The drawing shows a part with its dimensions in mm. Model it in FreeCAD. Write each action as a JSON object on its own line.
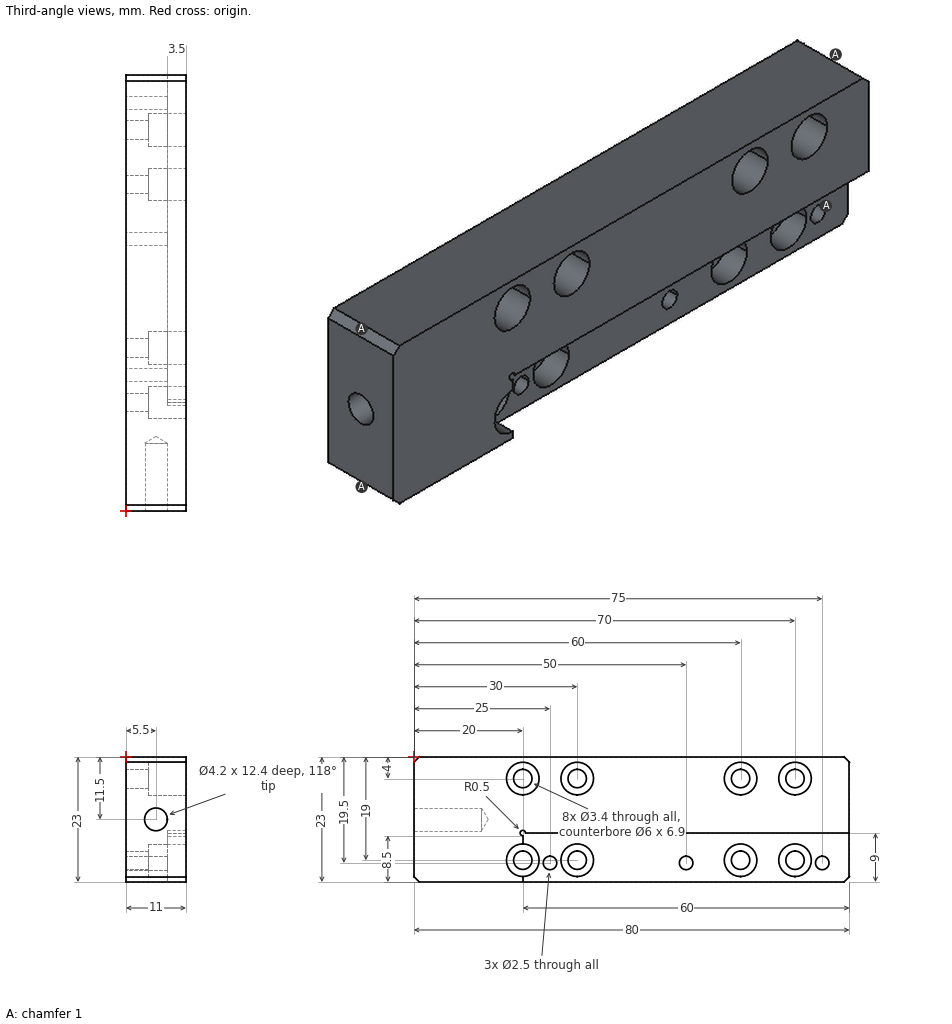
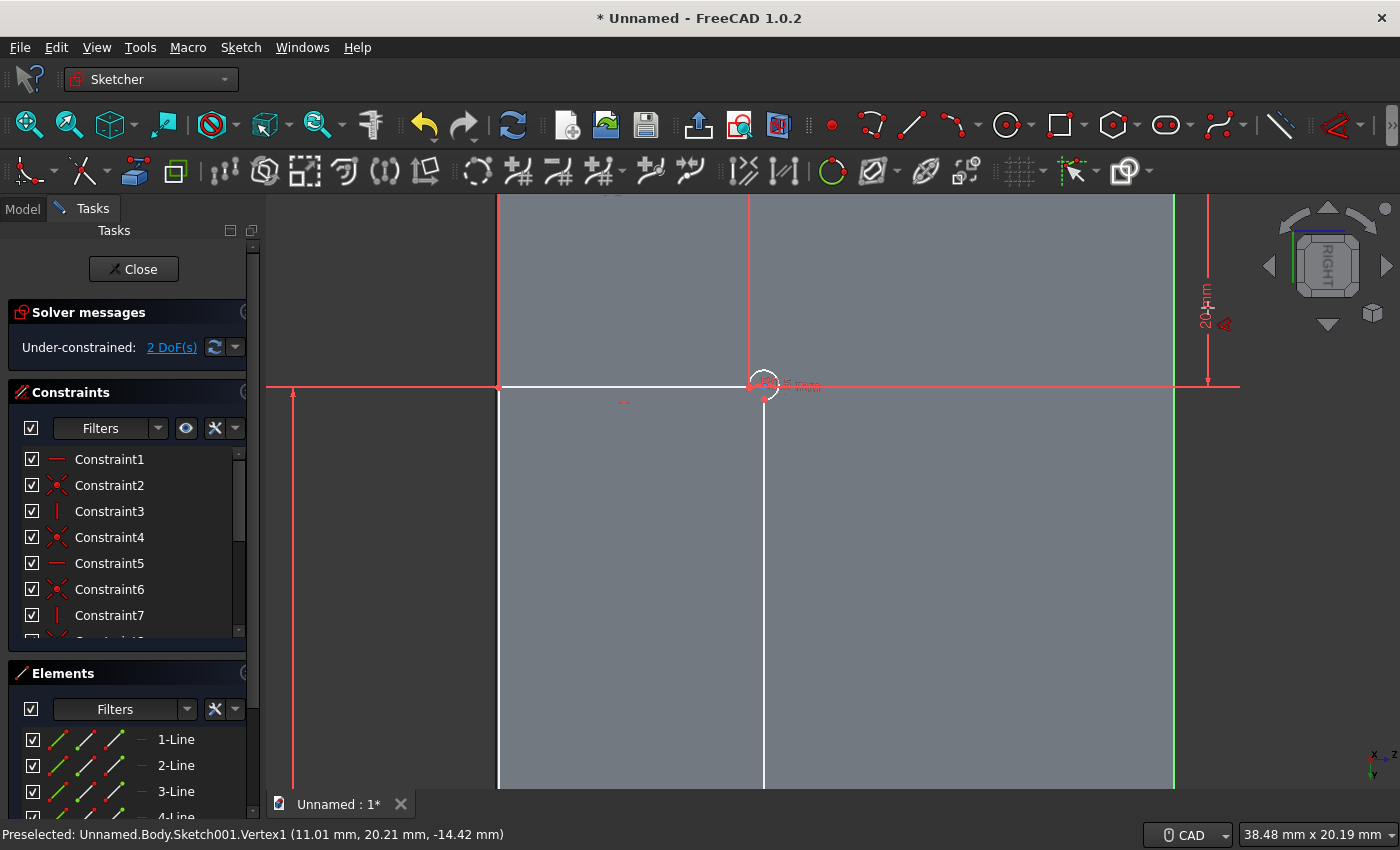
{"action": "scroll", "coordinate": [750, 395], "scroll_direction": "down", "scroll_amount": 9}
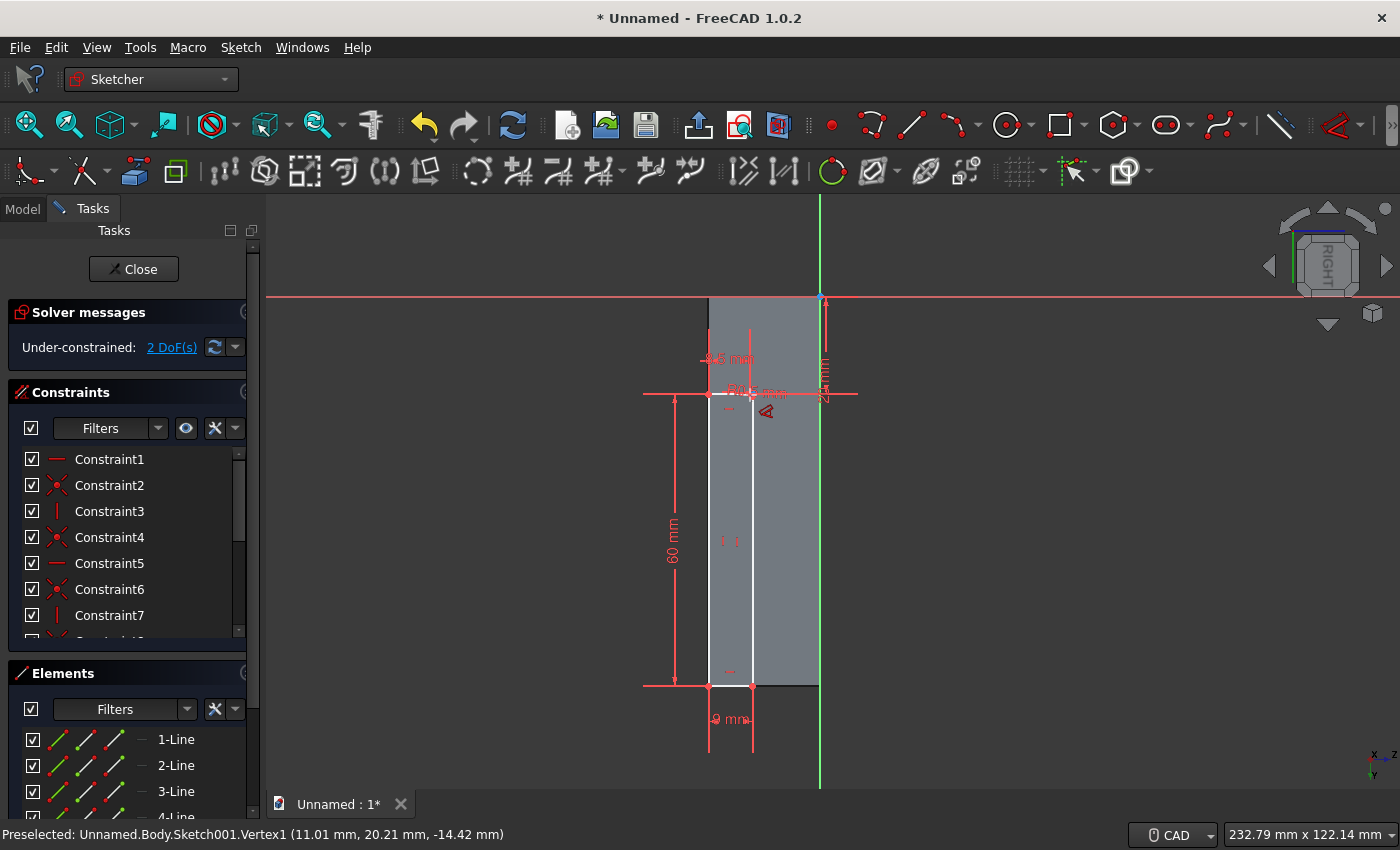
{"action": "left_click", "coordinate": [709, 394]}
{"action": "left_click", "coordinate": [765, 263]}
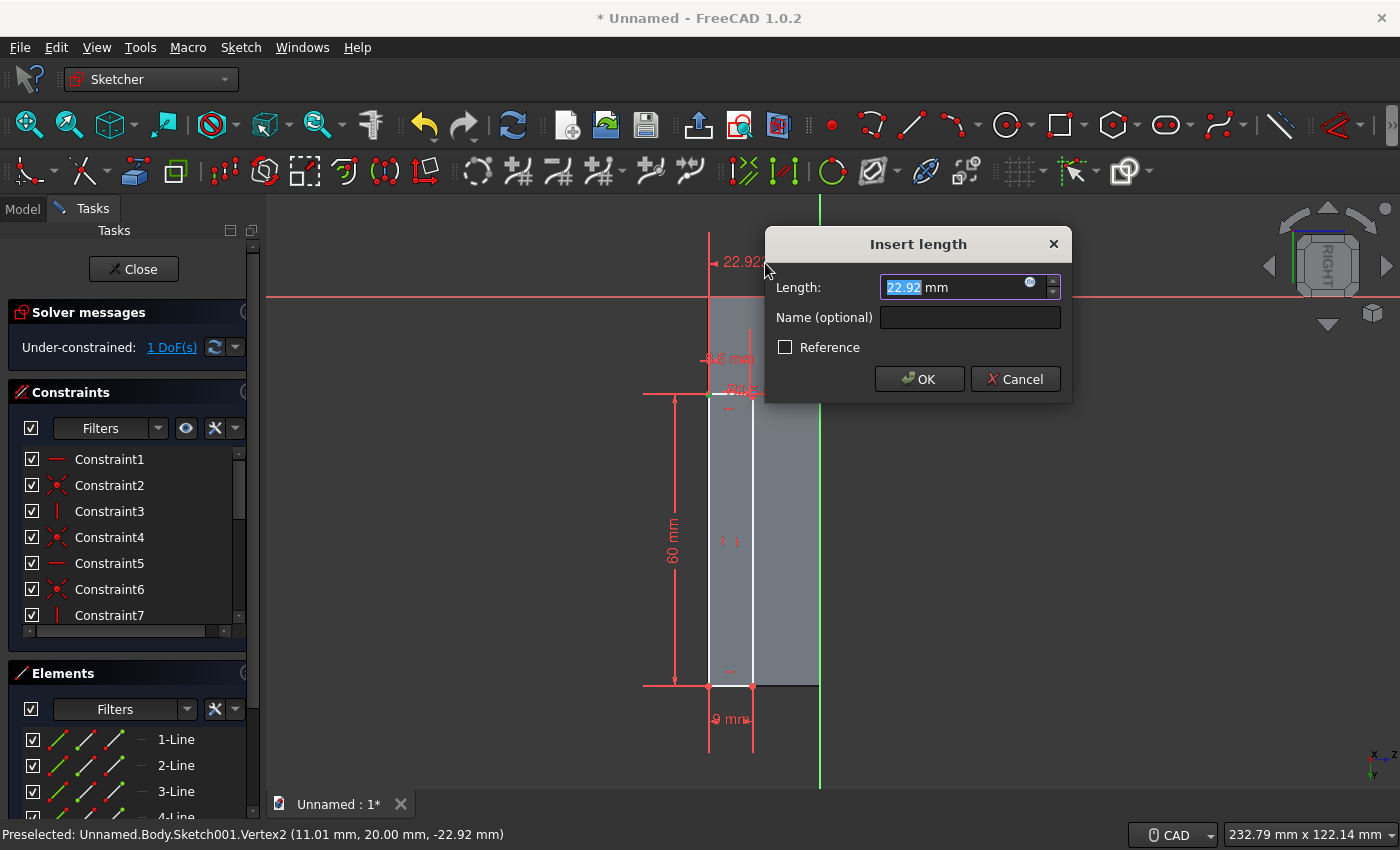
{"action": "type", "text": "23"}
{"action": "key", "text": "Return"}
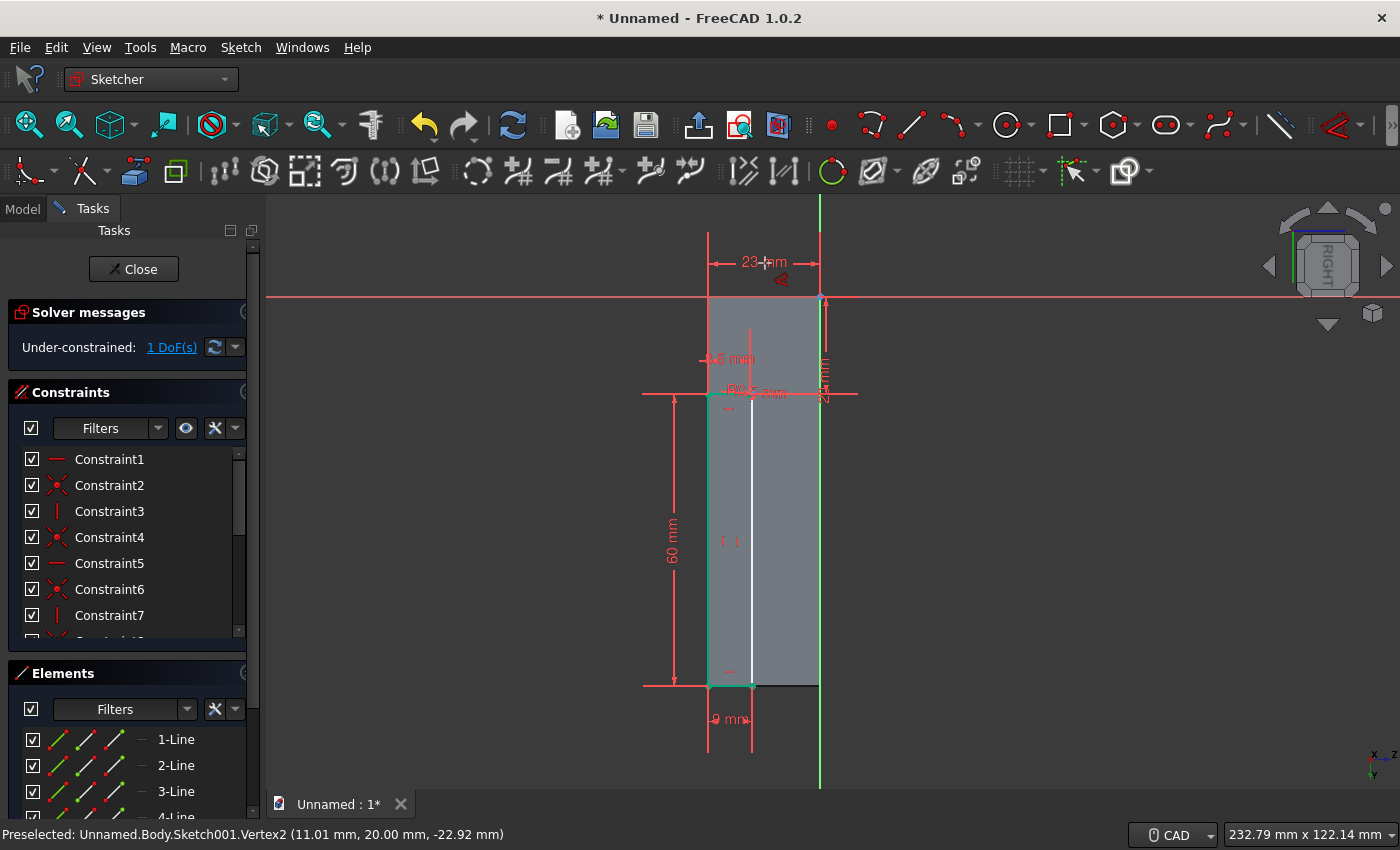
{"action": "scroll", "coordinate": [752, 394], "scroll_direction": "up", "scroll_amount": 9}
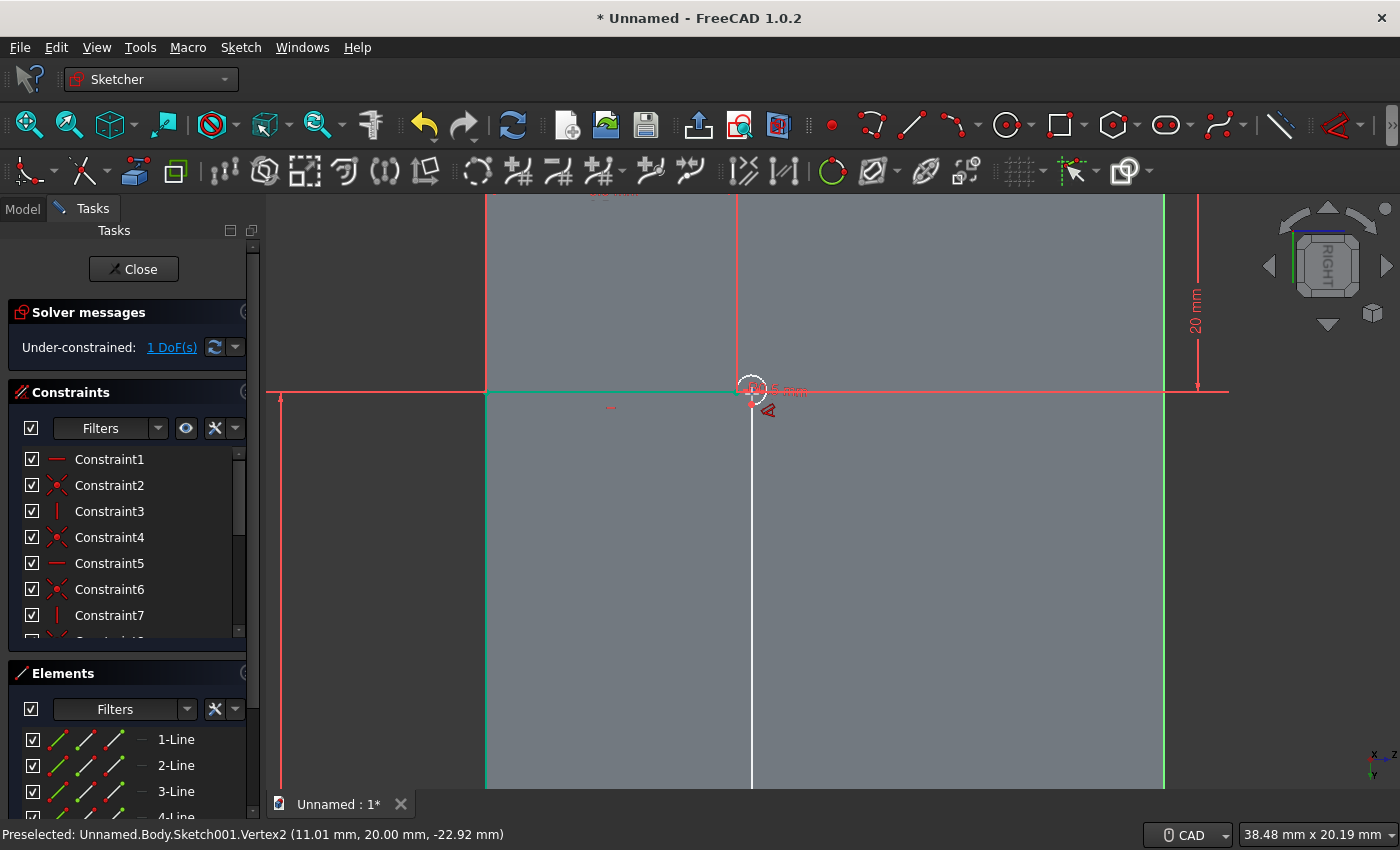
{"action": "left_click", "coordinate": [751, 390]}
{"action": "left_click", "coordinate": [1198, 267]}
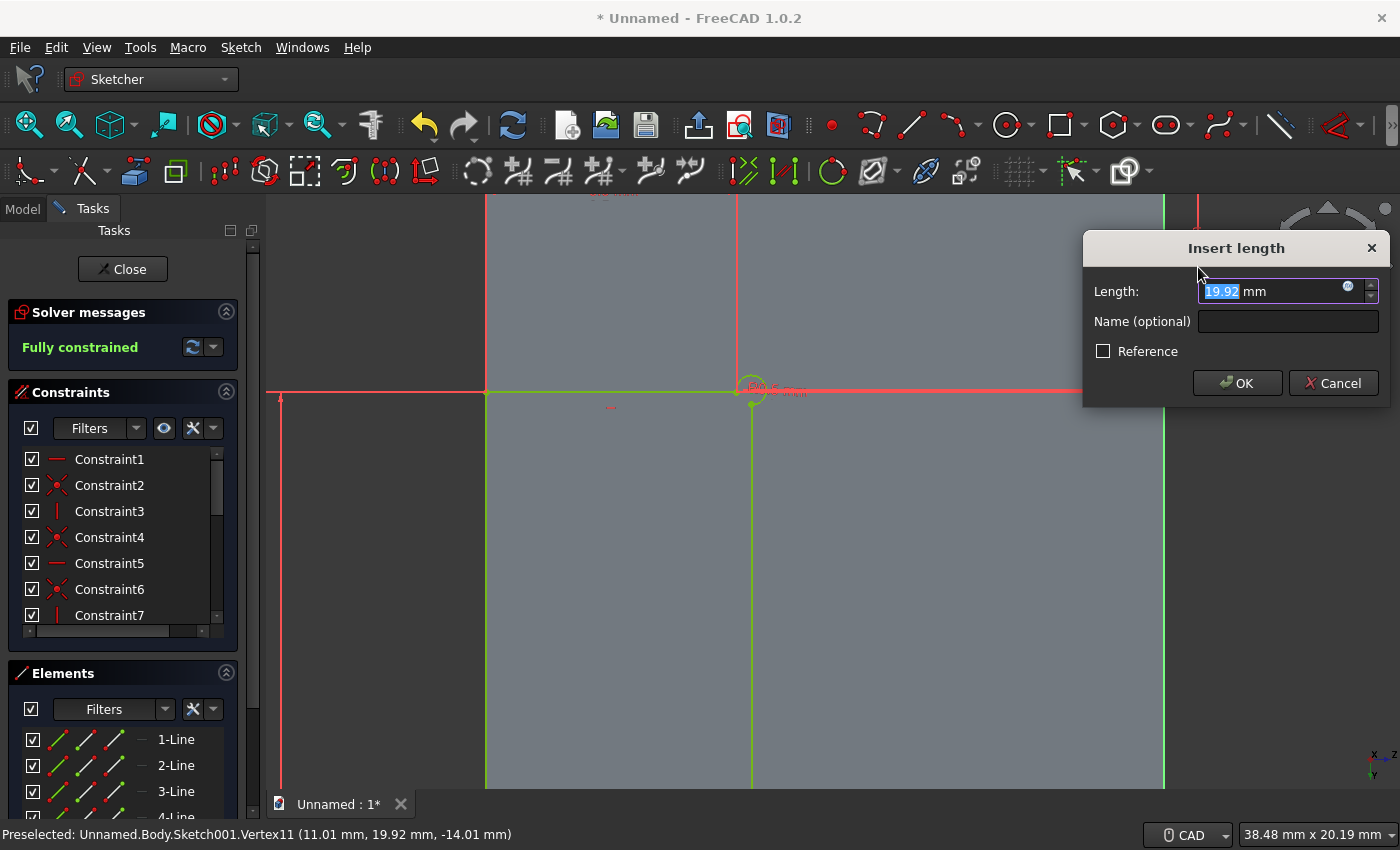
{"action": "type", "text": "20"}
{"action": "key", "text": "Return"}
{"action": "key", "text": "Escape"}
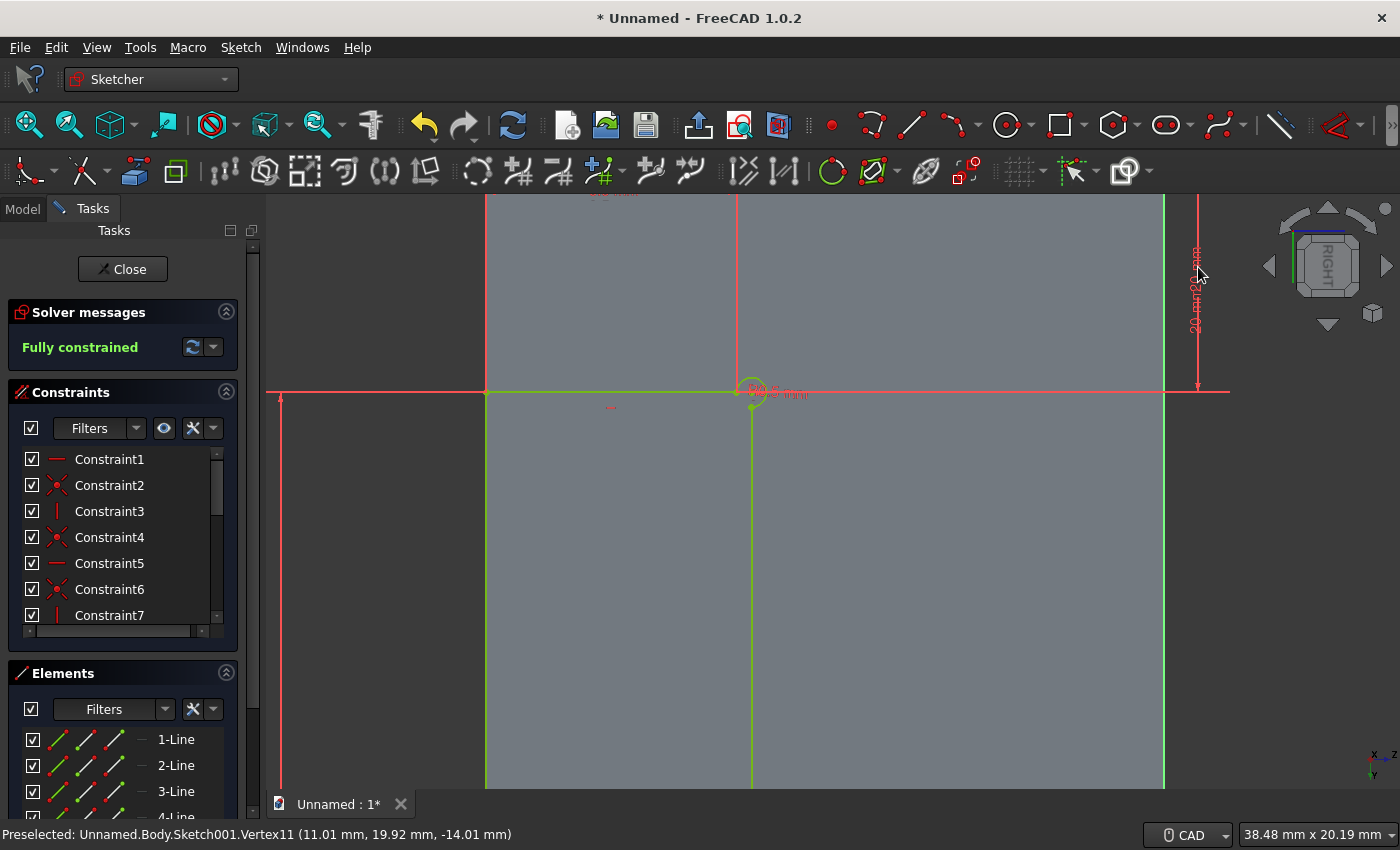
{"action": "left_click", "coordinate": [123, 269]}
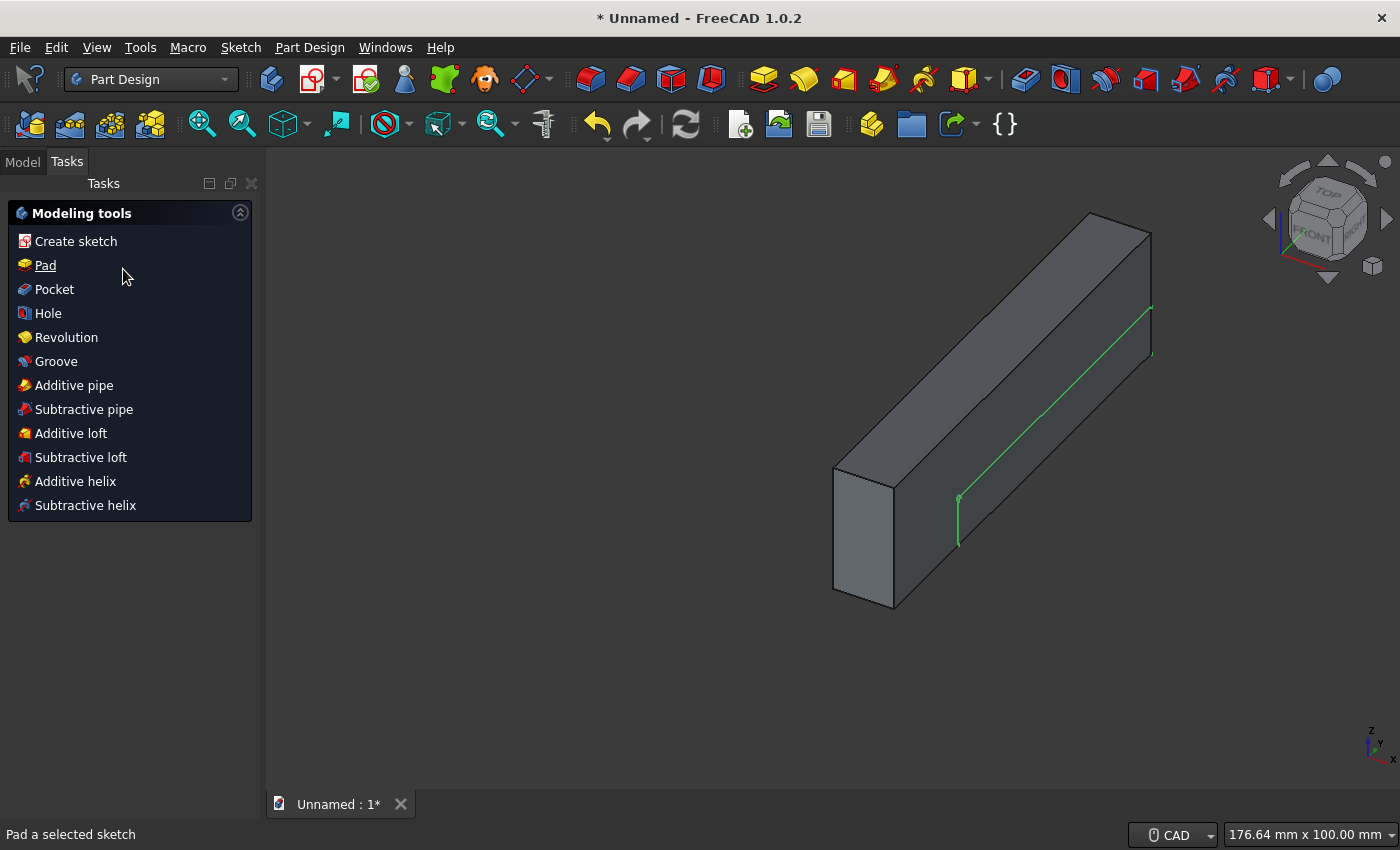
{"action": "left_click", "coordinate": [1026, 80]}